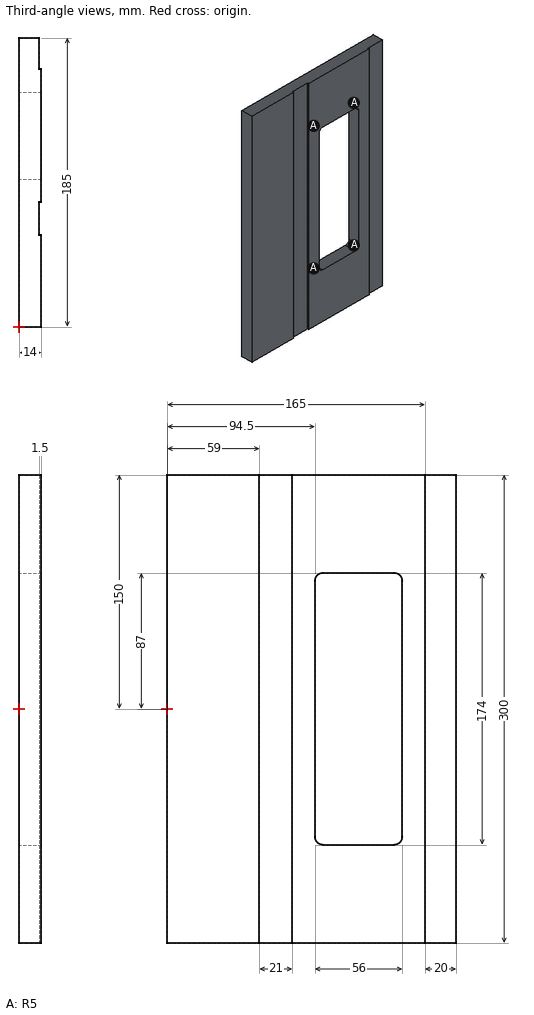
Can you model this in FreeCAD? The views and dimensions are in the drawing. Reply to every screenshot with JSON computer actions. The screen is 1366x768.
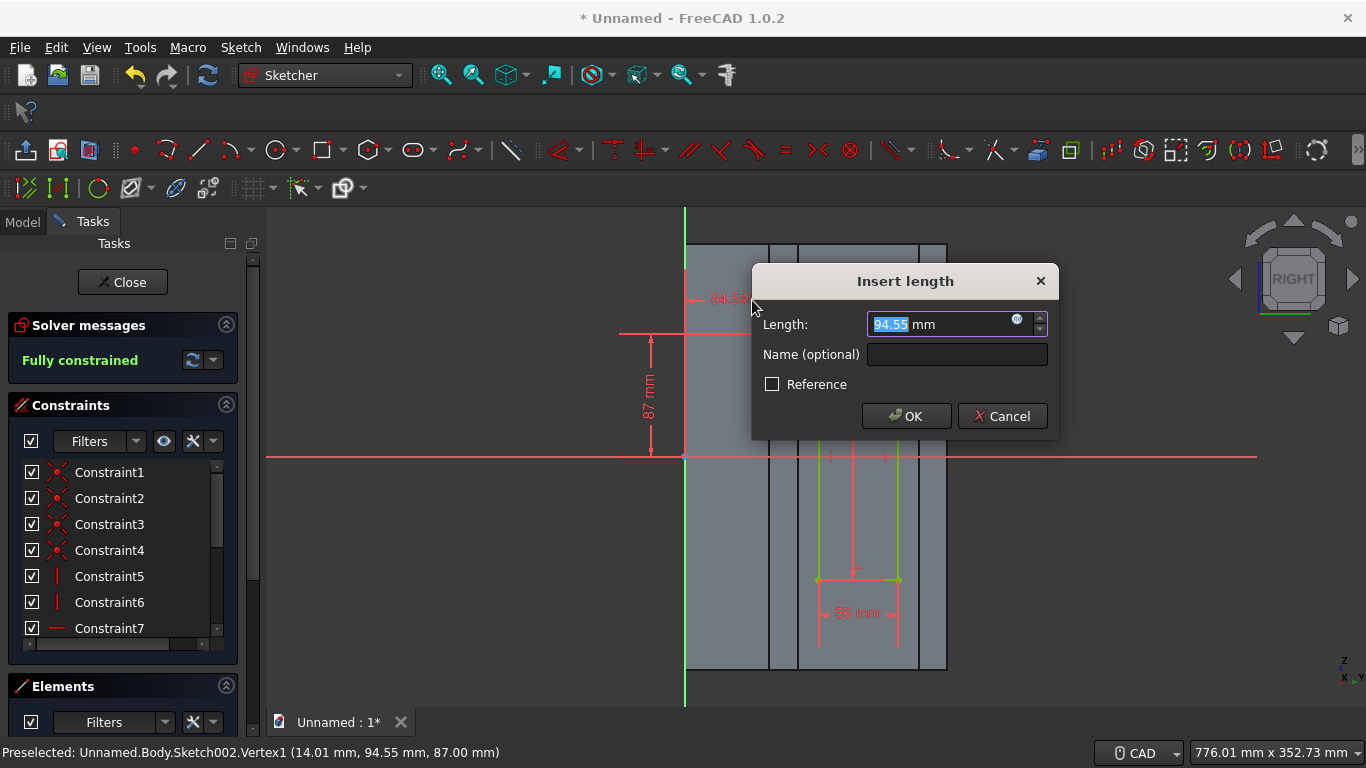
{"action": "type", "text": "94.5"}
{"action": "key", "text": "Return"}
{"action": "key", "text": "Escape"}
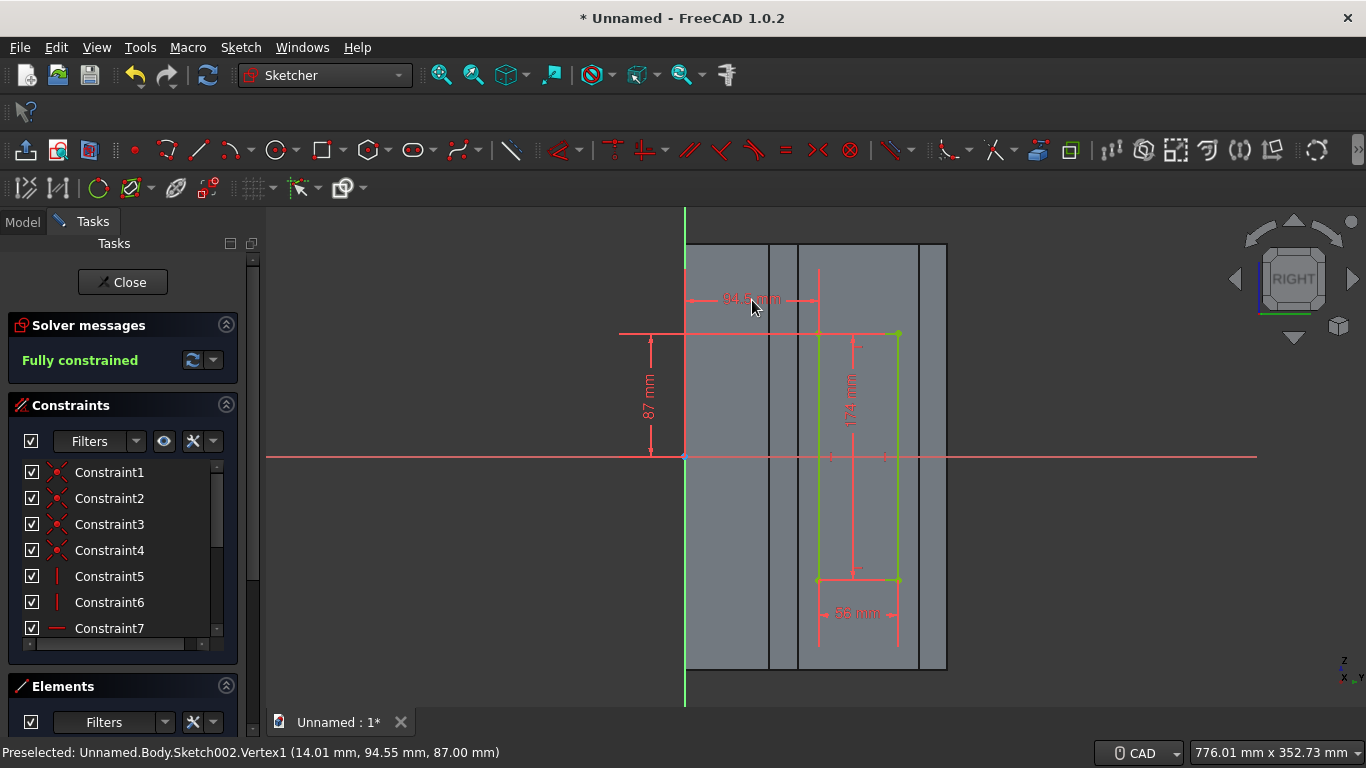
{"action": "left_click", "coordinate": [123, 282]}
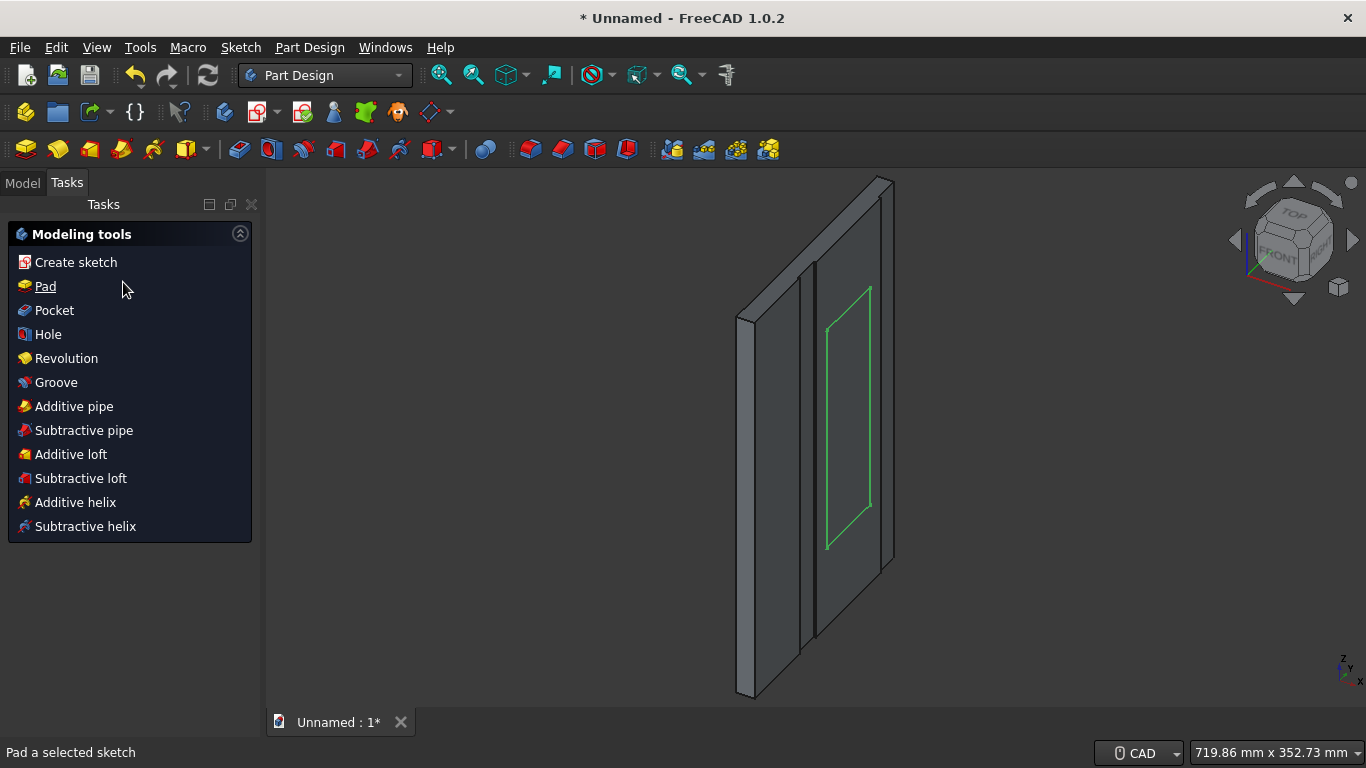
{"action": "left_click", "coordinate": [240, 150]}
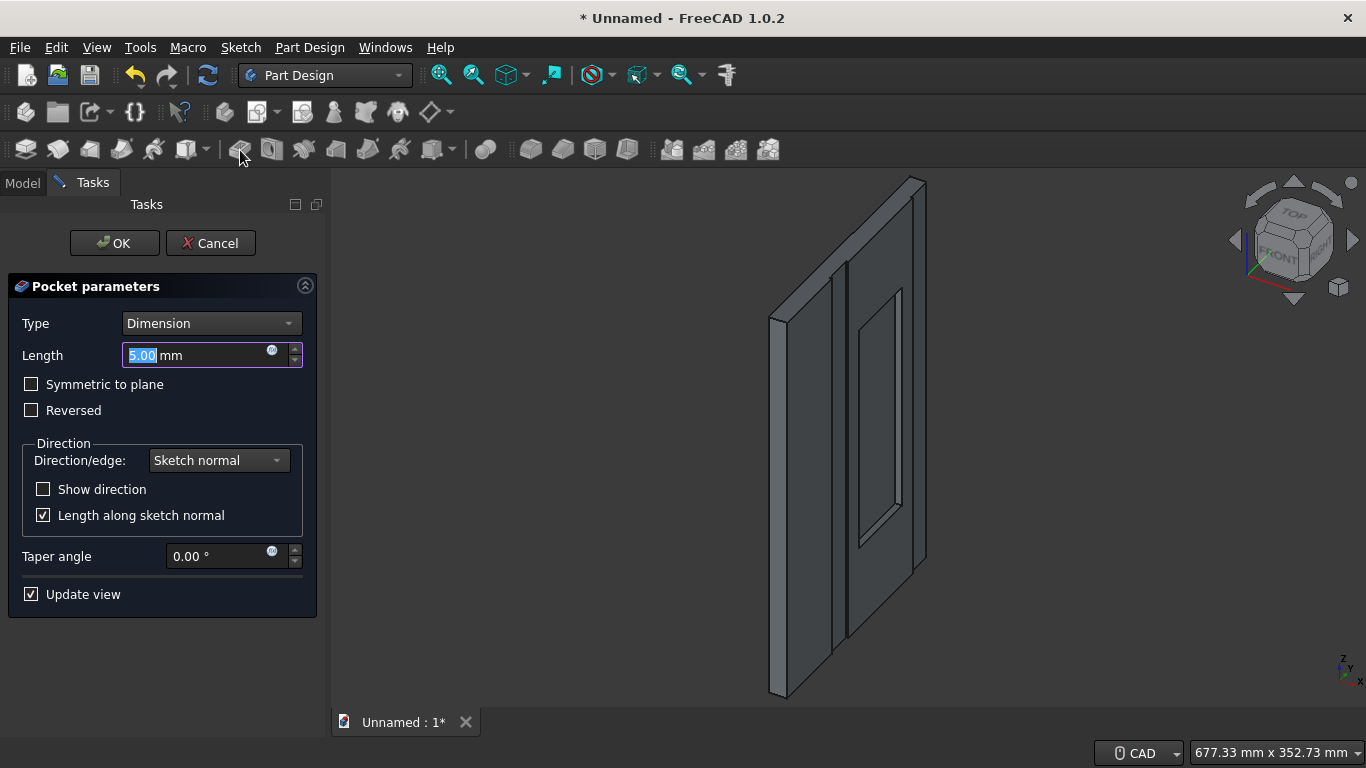
{"action": "left_click", "coordinate": [212, 324]}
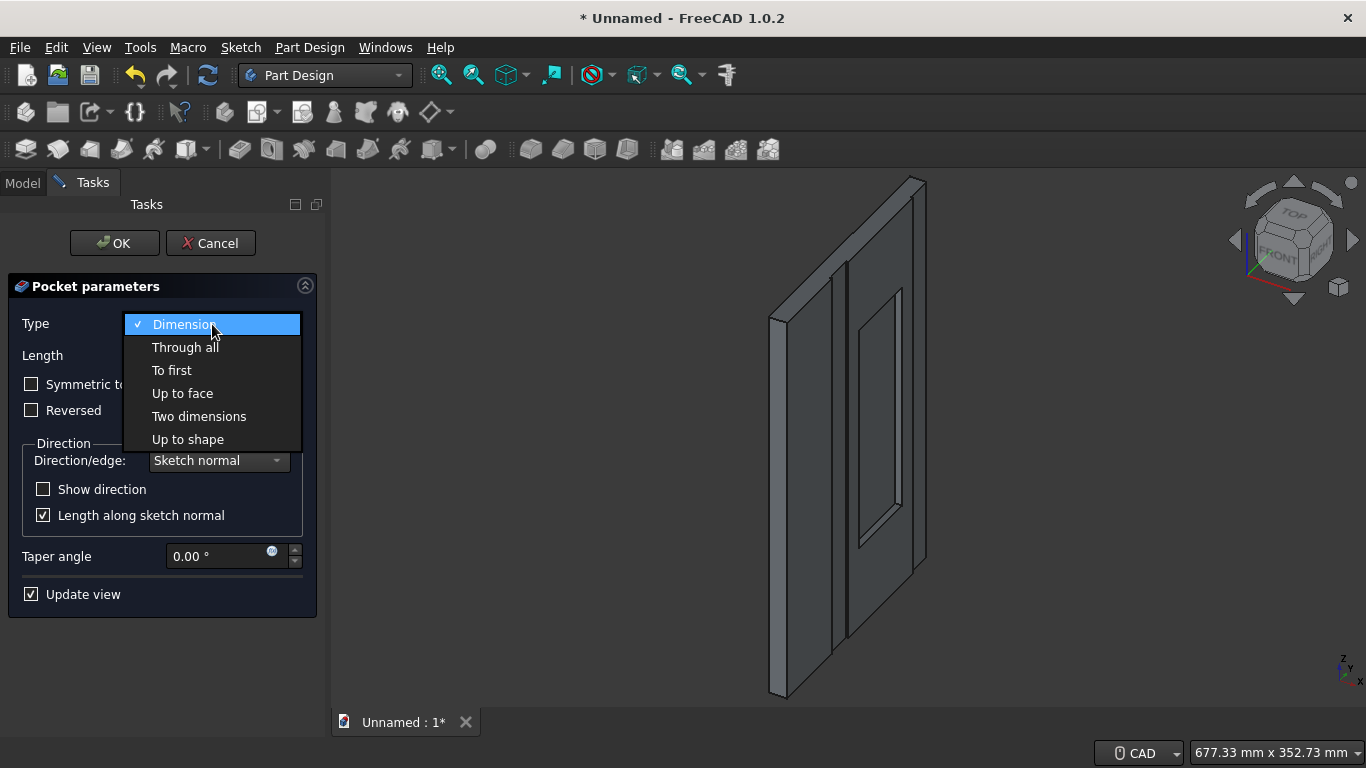
{"action": "left_click", "coordinate": [212, 370]}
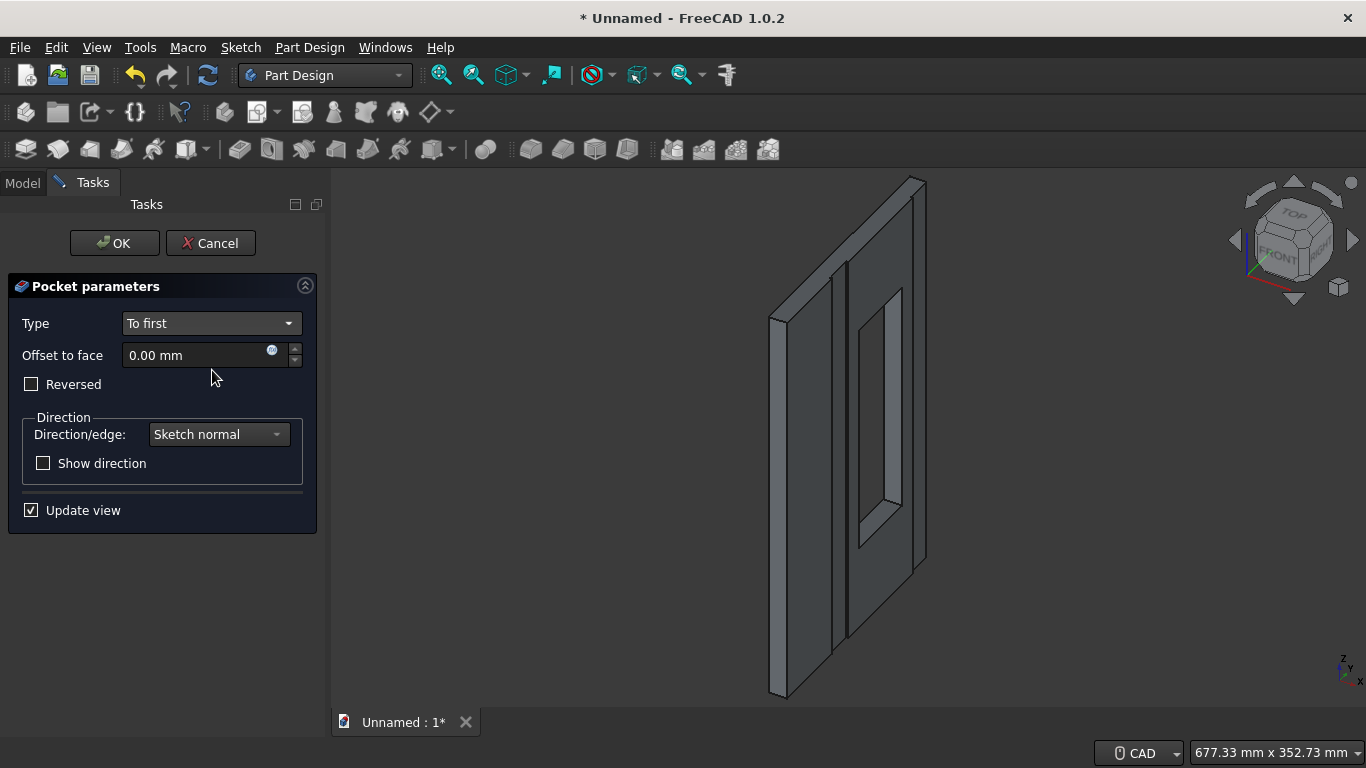
{"action": "left_click", "coordinate": [115, 243]}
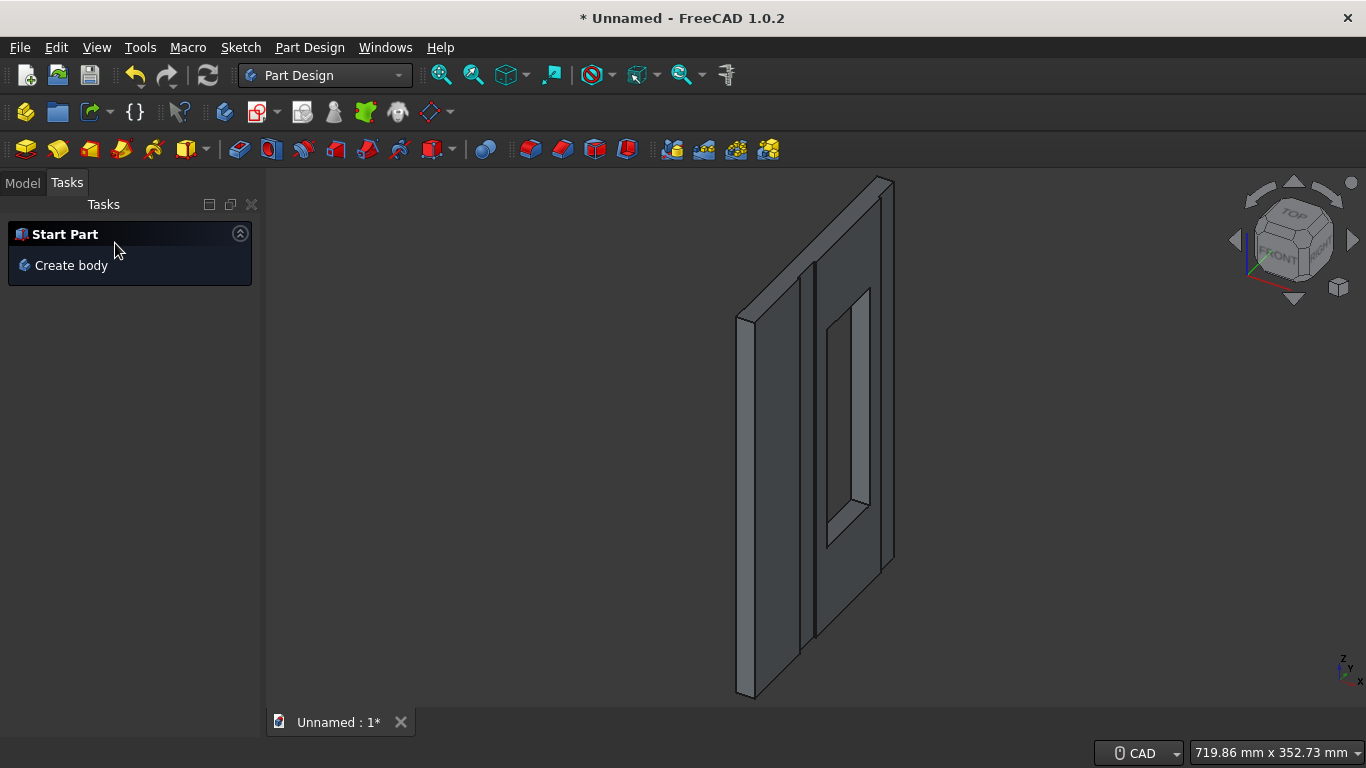
{"action": "scroll", "coordinate": [860, 501], "scroll_direction": "up", "scroll_amount": 4}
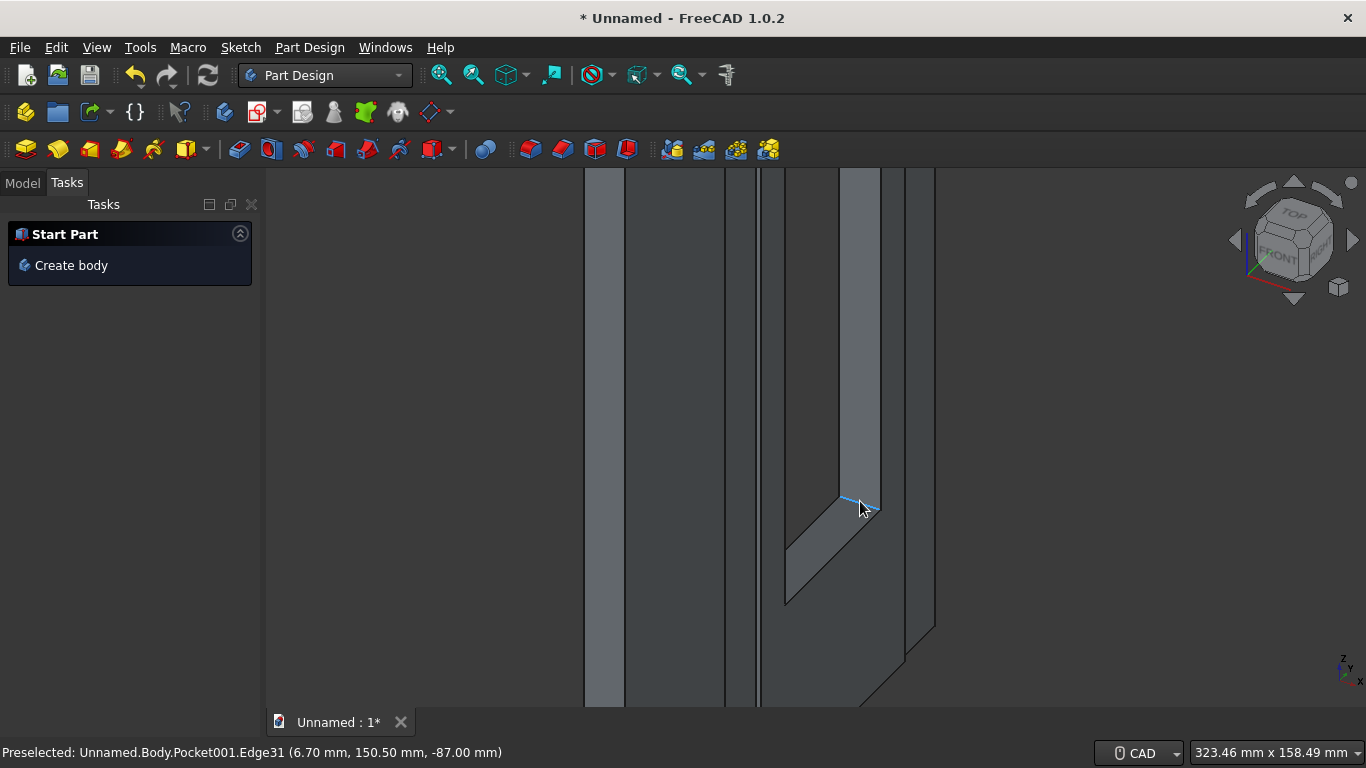
{"action": "left_click", "coordinate": [442, 76]}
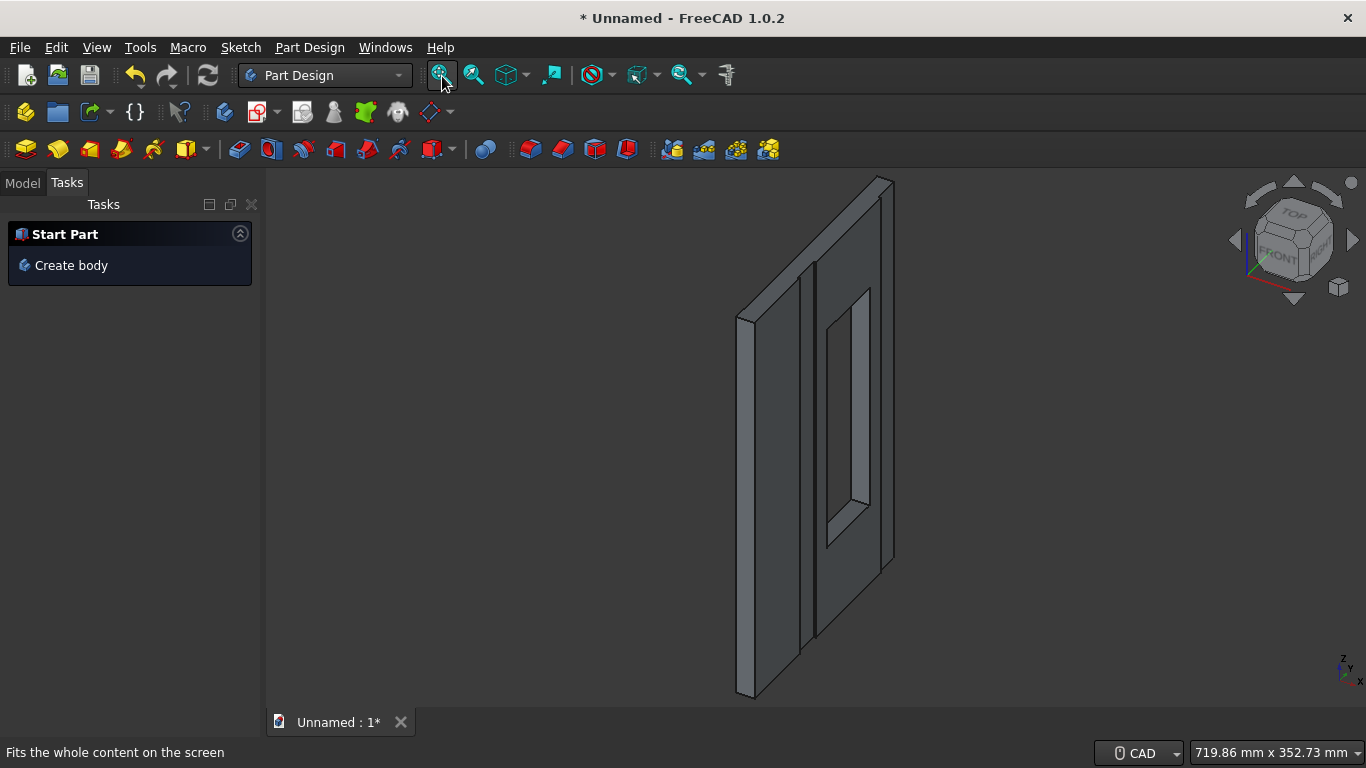
{"action": "key", "text": "0"}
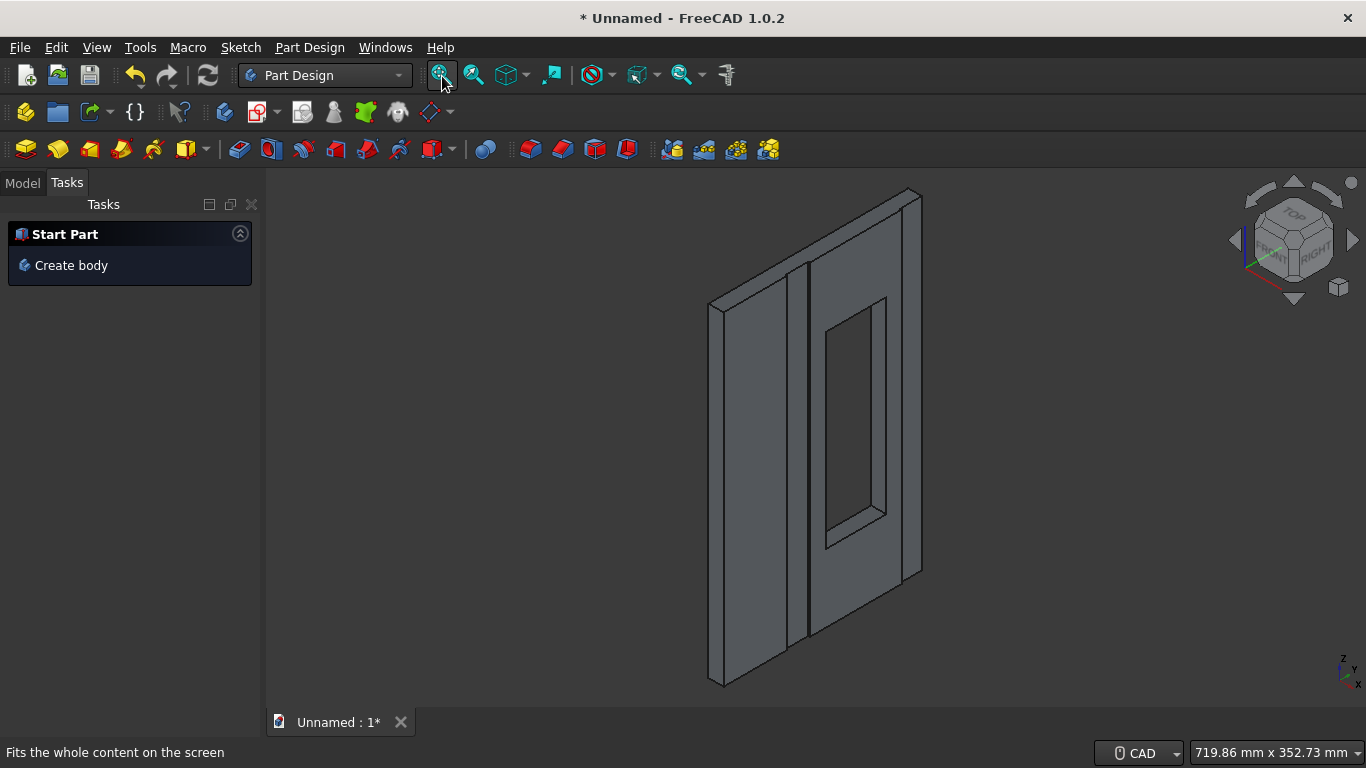
{"action": "scroll", "coordinate": [879, 509], "scroll_direction": "up", "scroll_amount": 4}